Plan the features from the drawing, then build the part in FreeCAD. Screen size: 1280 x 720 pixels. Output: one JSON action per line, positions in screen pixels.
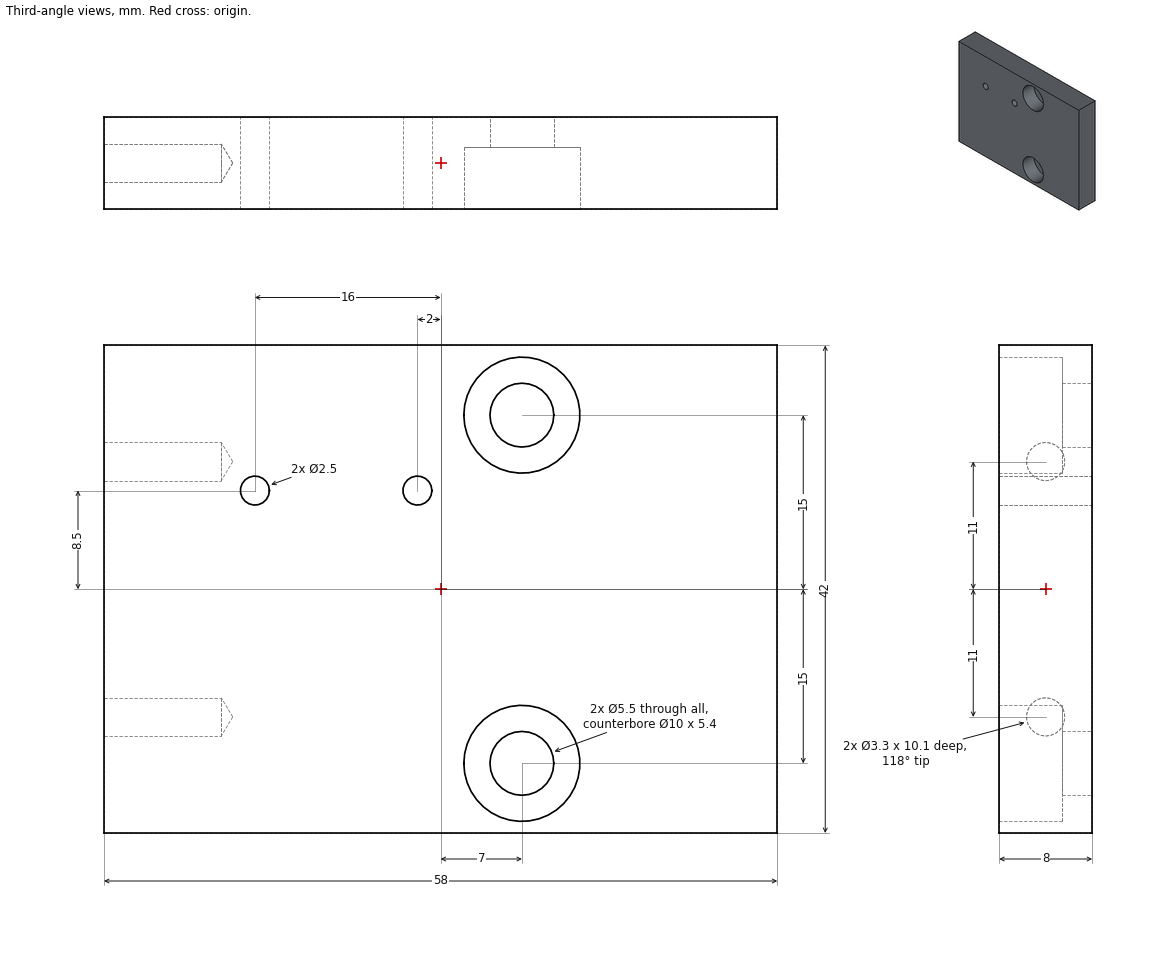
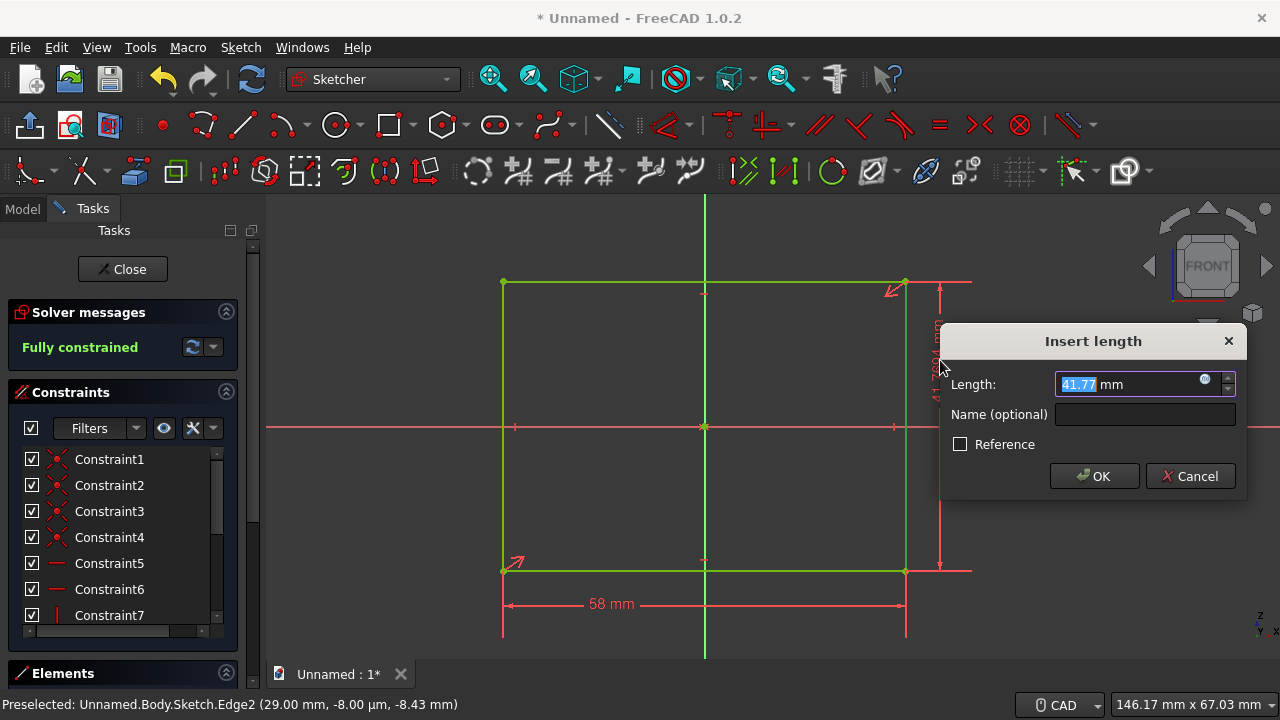
{"action": "type", "text": "42"}
{"action": "key", "text": "Return"}
{"action": "key", "text": "Escape"}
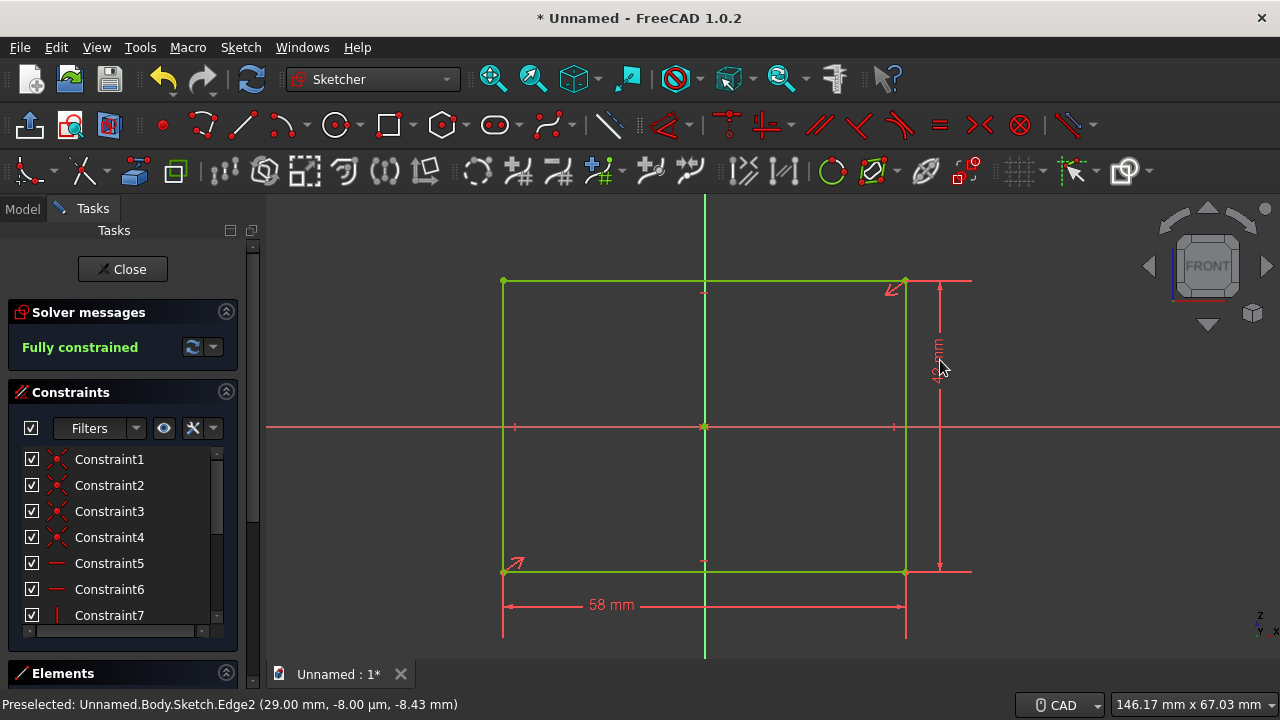
{"action": "left_click", "coordinate": [123, 269]}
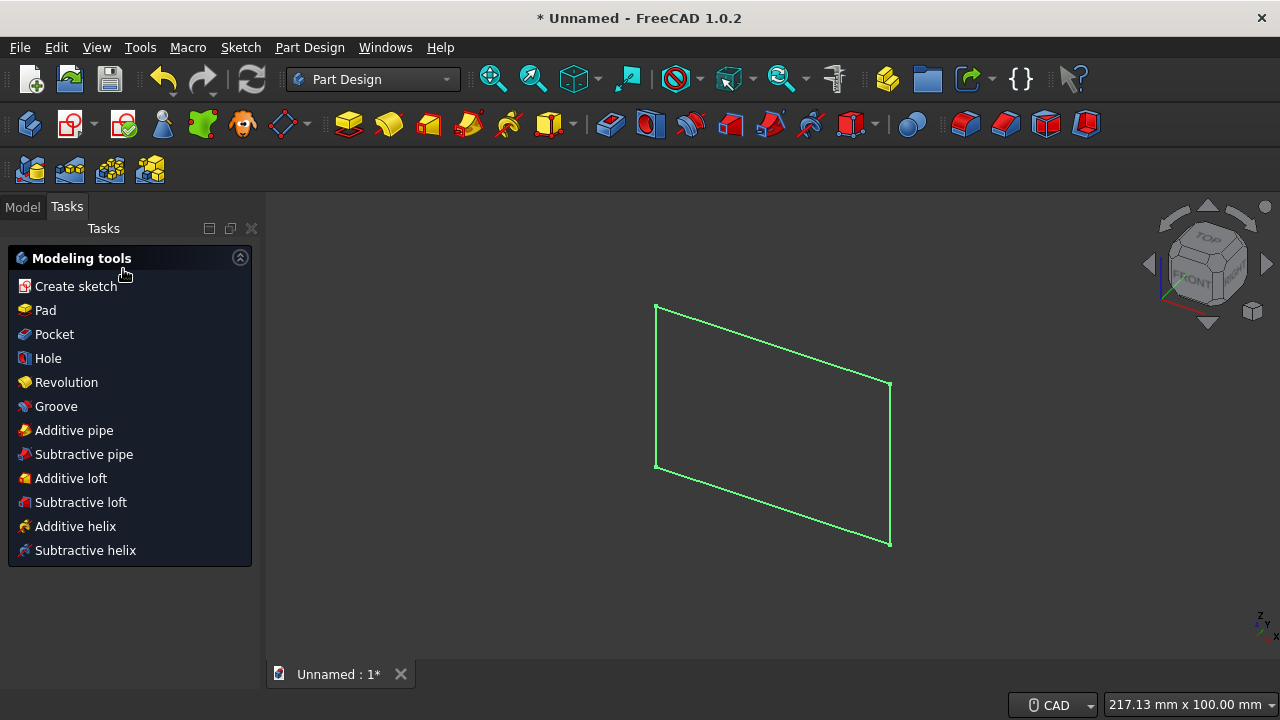
{"action": "left_click", "coordinate": [350, 124]}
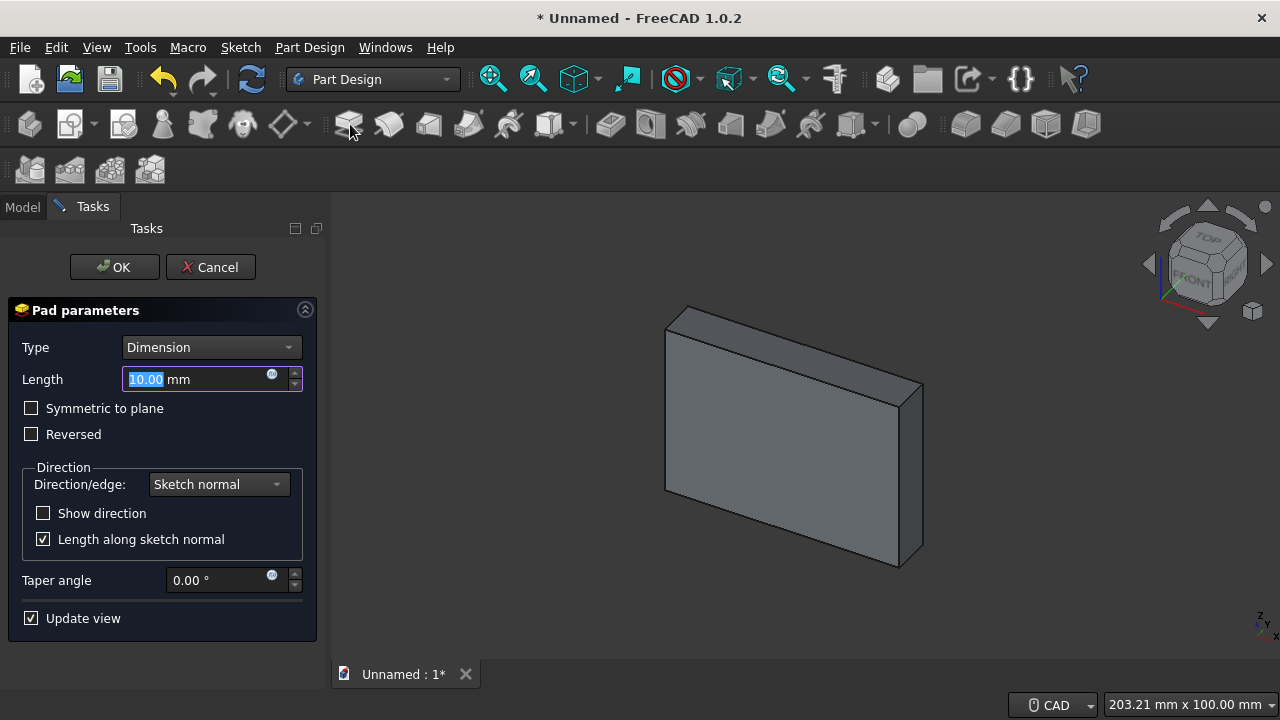
{"action": "type", "text": "8"}
{"action": "key", "text": "Tab"}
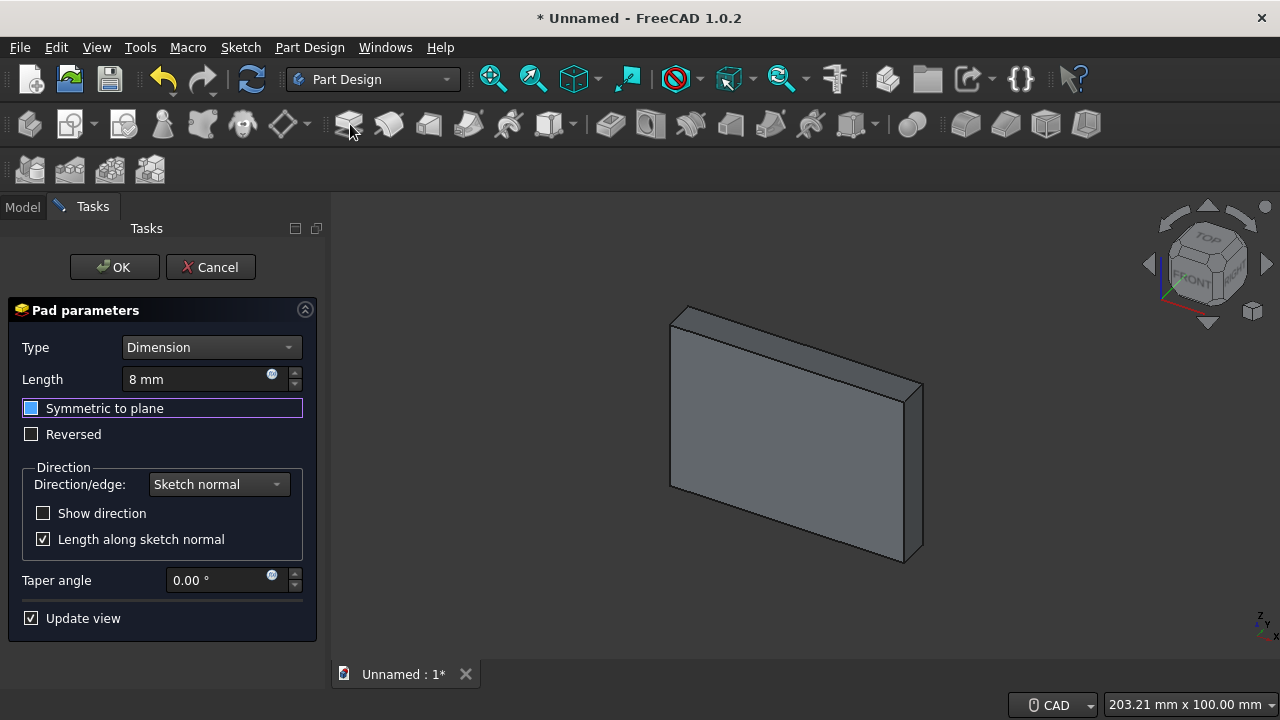
{"action": "left_click", "coordinate": [30, 408]}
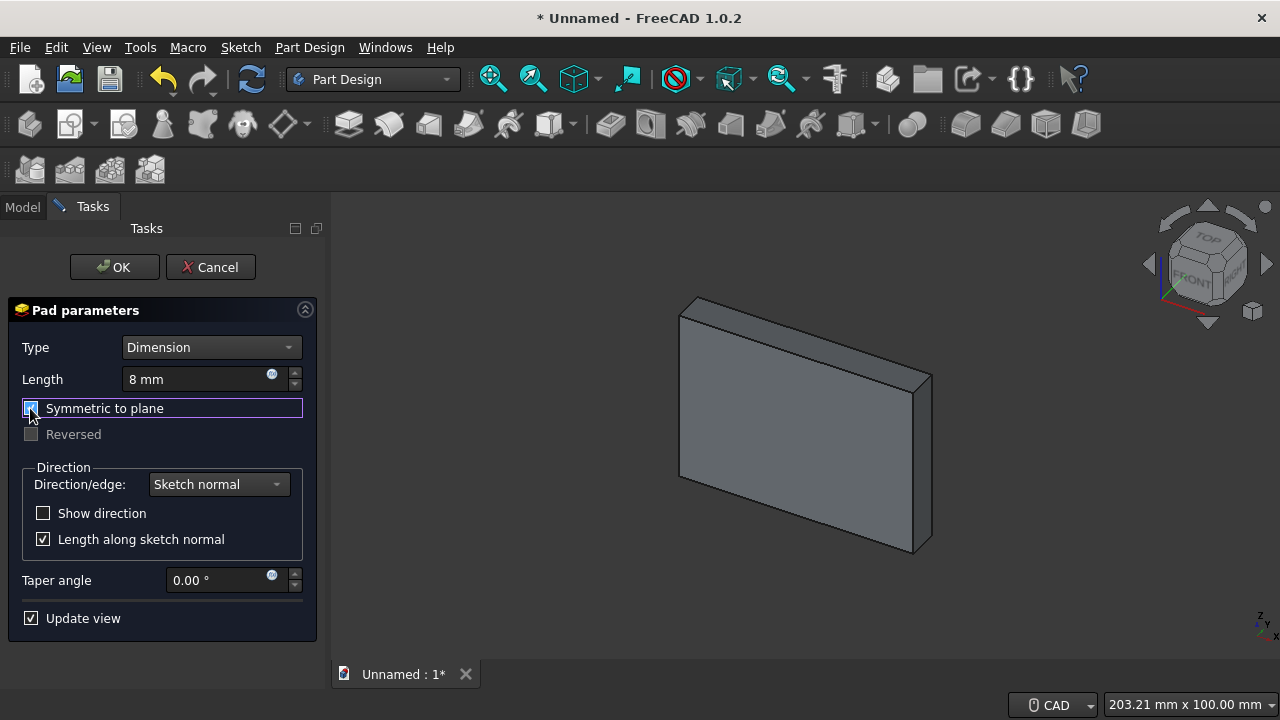
{"action": "left_click", "coordinate": [115, 267]}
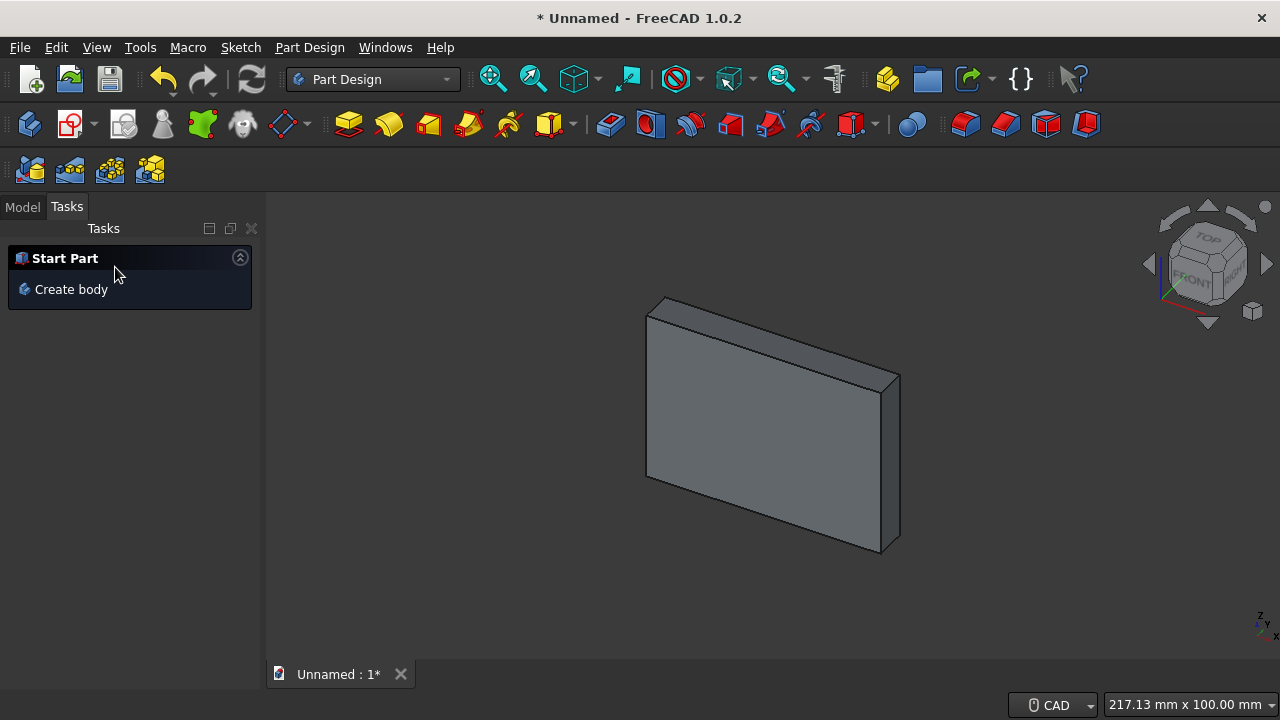
{"action": "left_click", "coordinate": [764, 434]}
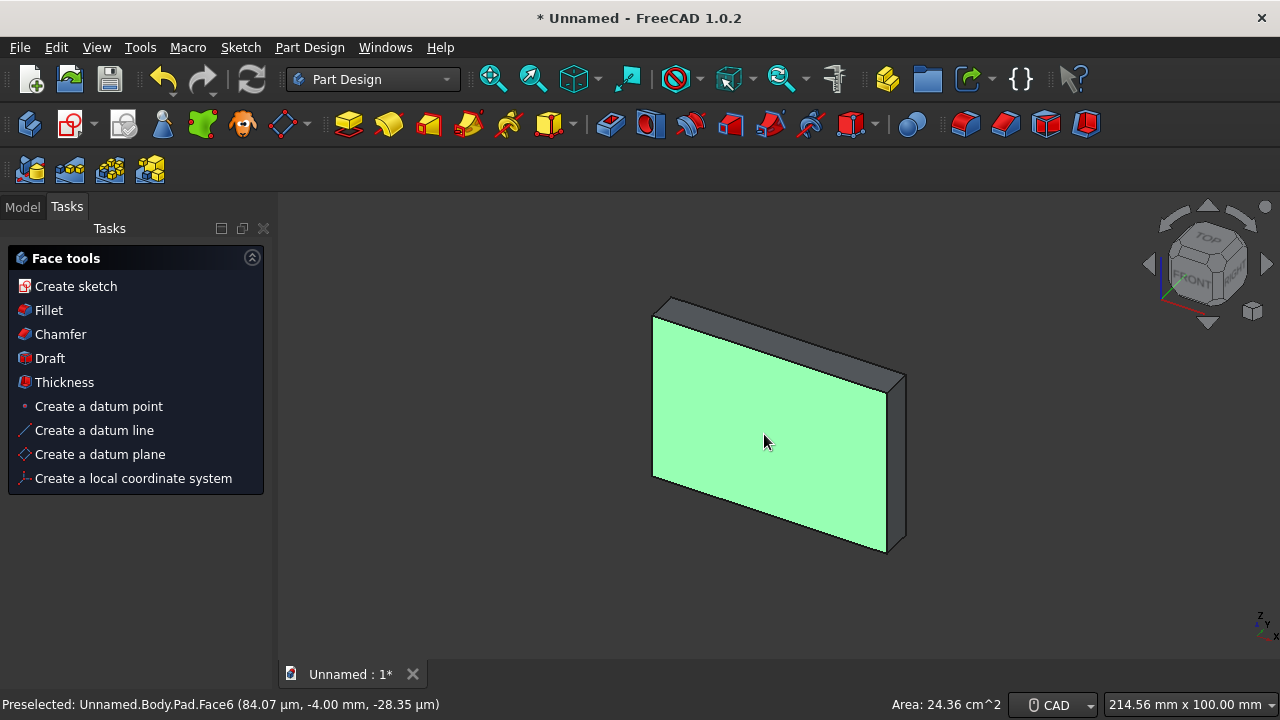
{"action": "left_click", "coordinate": [70, 124]}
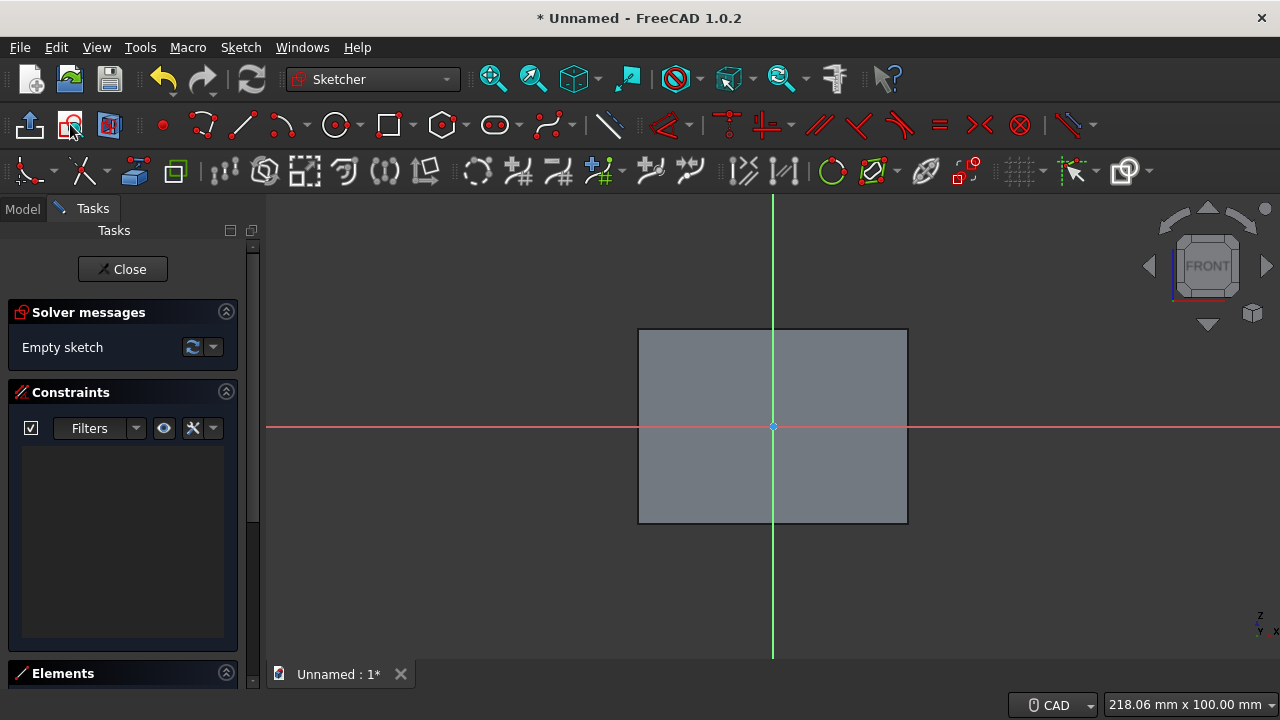
{"action": "scroll", "coordinate": [907, 426], "scroll_direction": "up", "scroll_amount": 3}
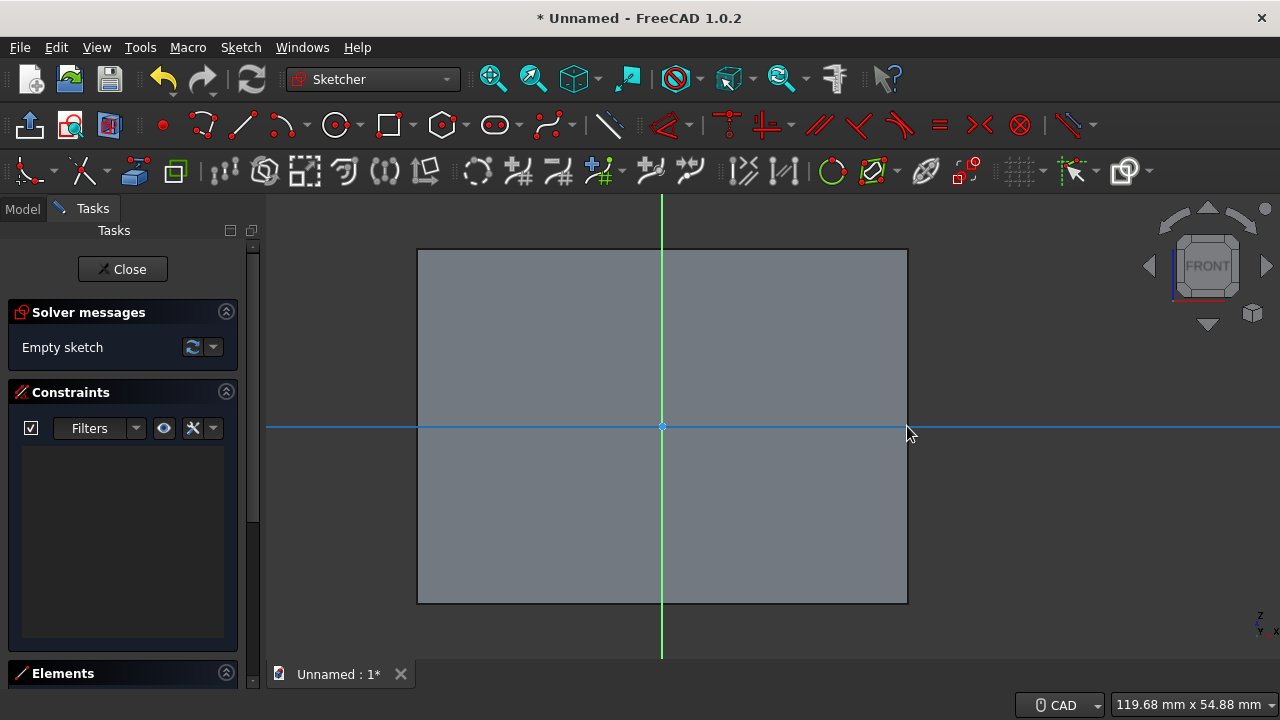
{"action": "left_click", "coordinate": [336, 126]}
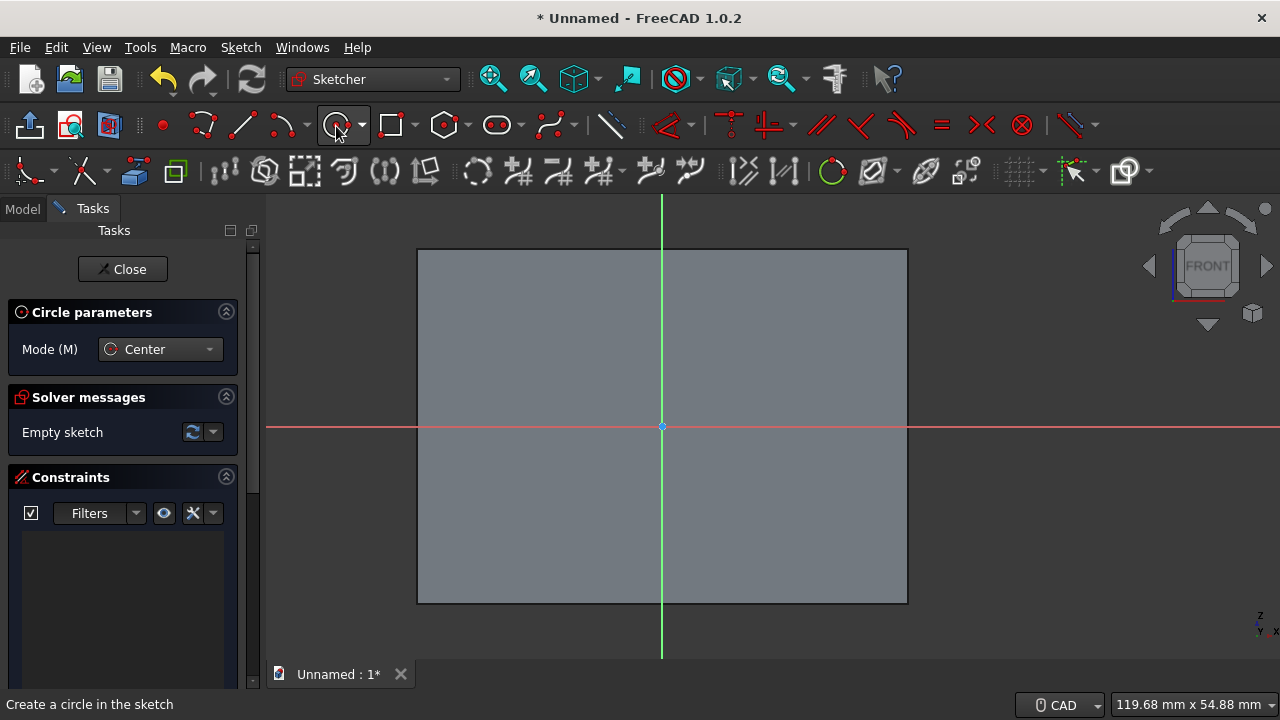
{"action": "left_click", "coordinate": [722, 554]}
{"action": "left_click", "coordinate": [738, 537]}